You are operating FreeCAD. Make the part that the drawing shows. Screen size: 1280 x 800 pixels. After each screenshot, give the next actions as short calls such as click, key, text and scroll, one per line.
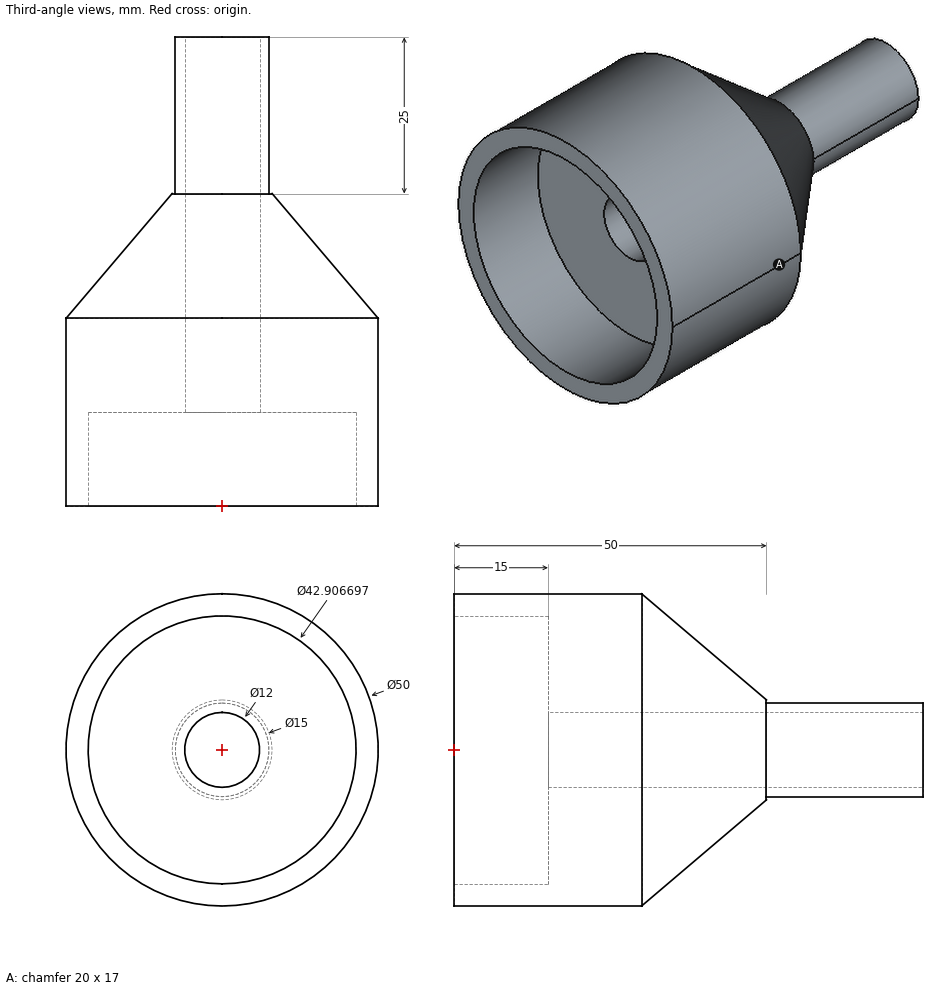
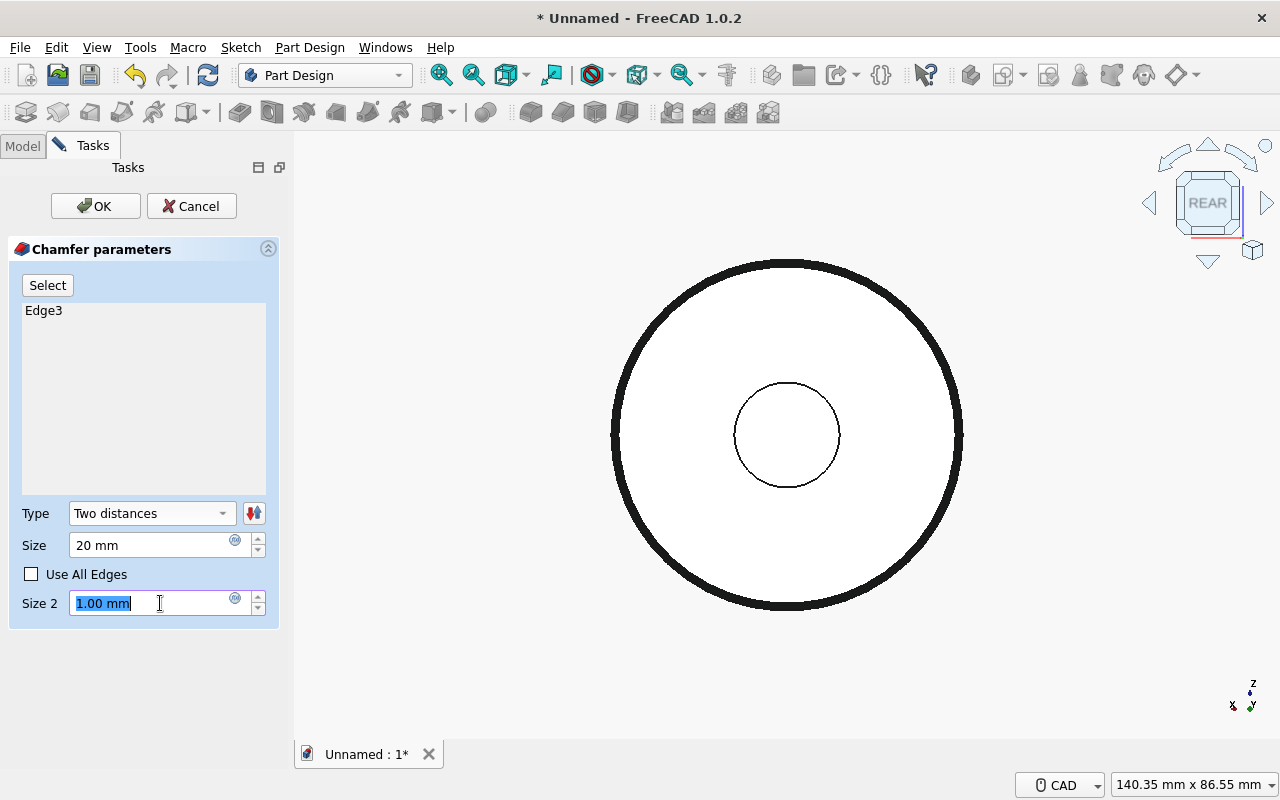
text(17)
key(Tab)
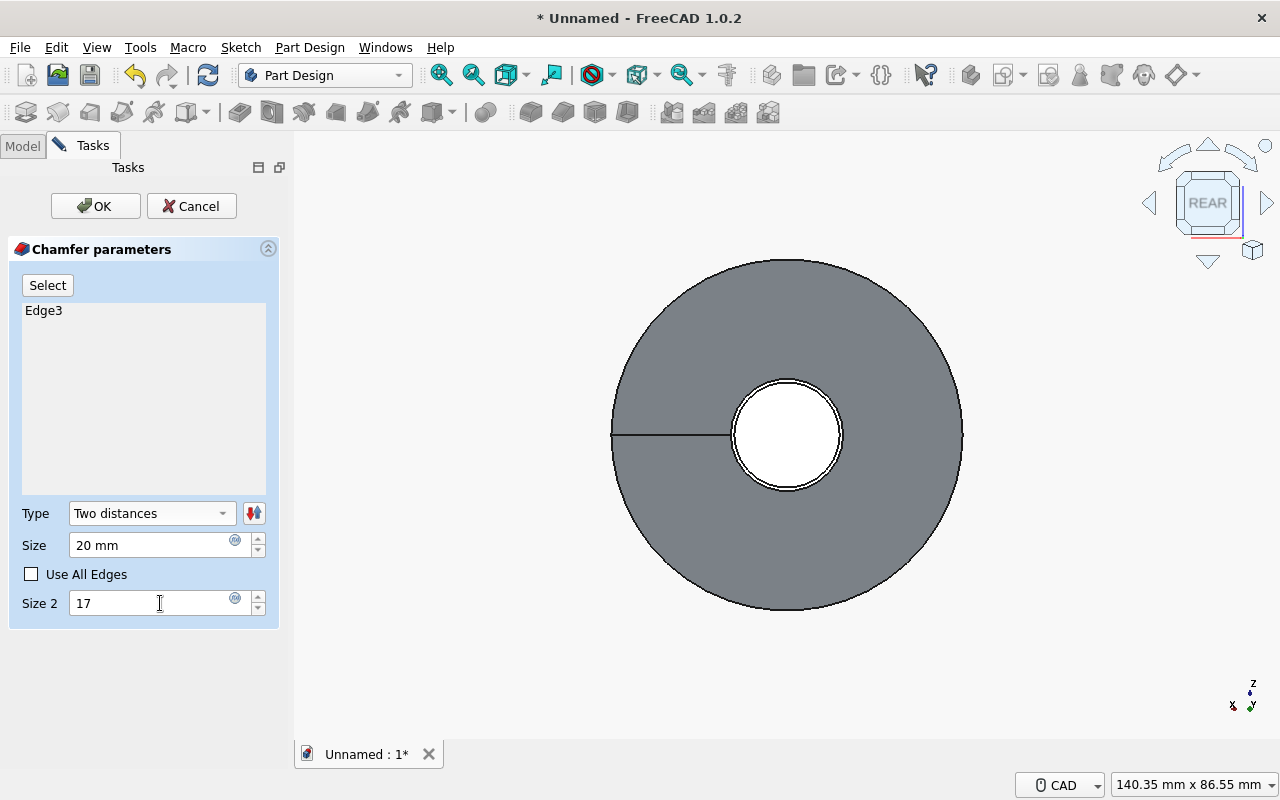
click(96, 206)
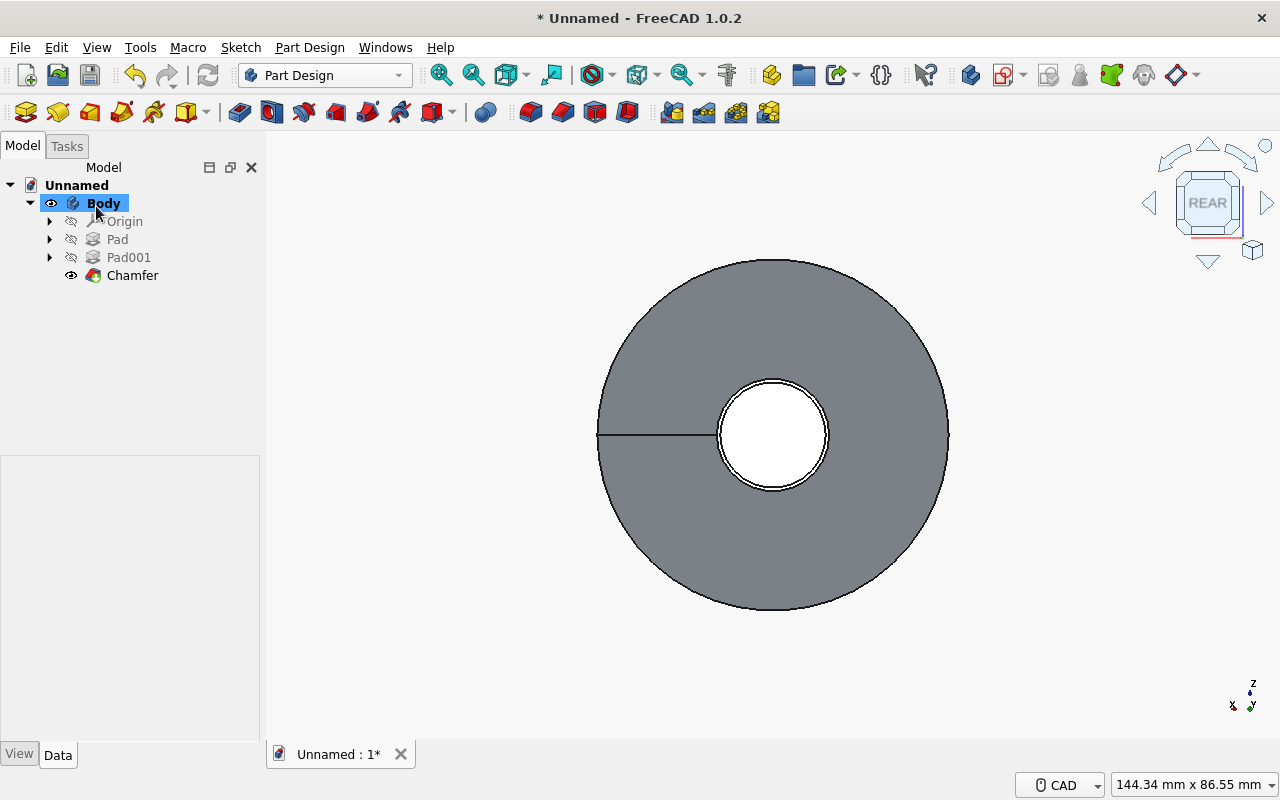
click(773, 434)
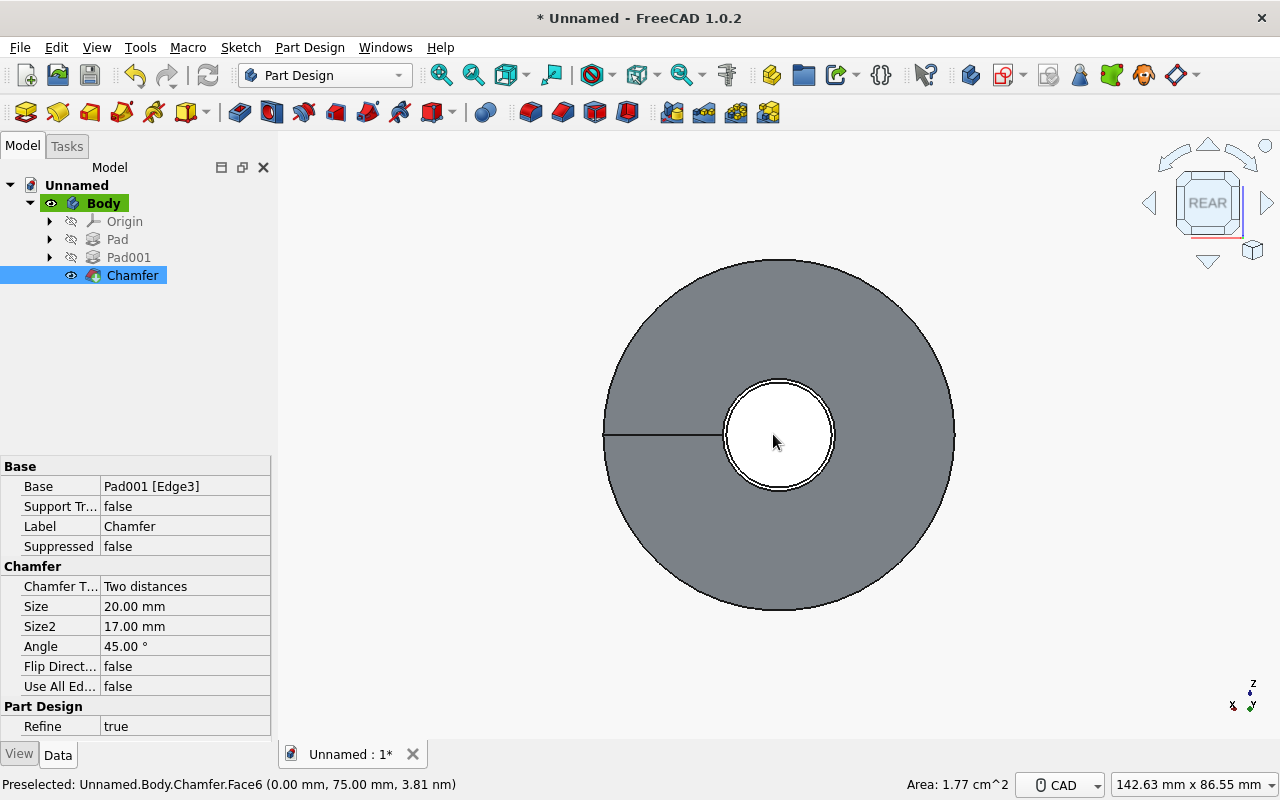
click(1004, 76)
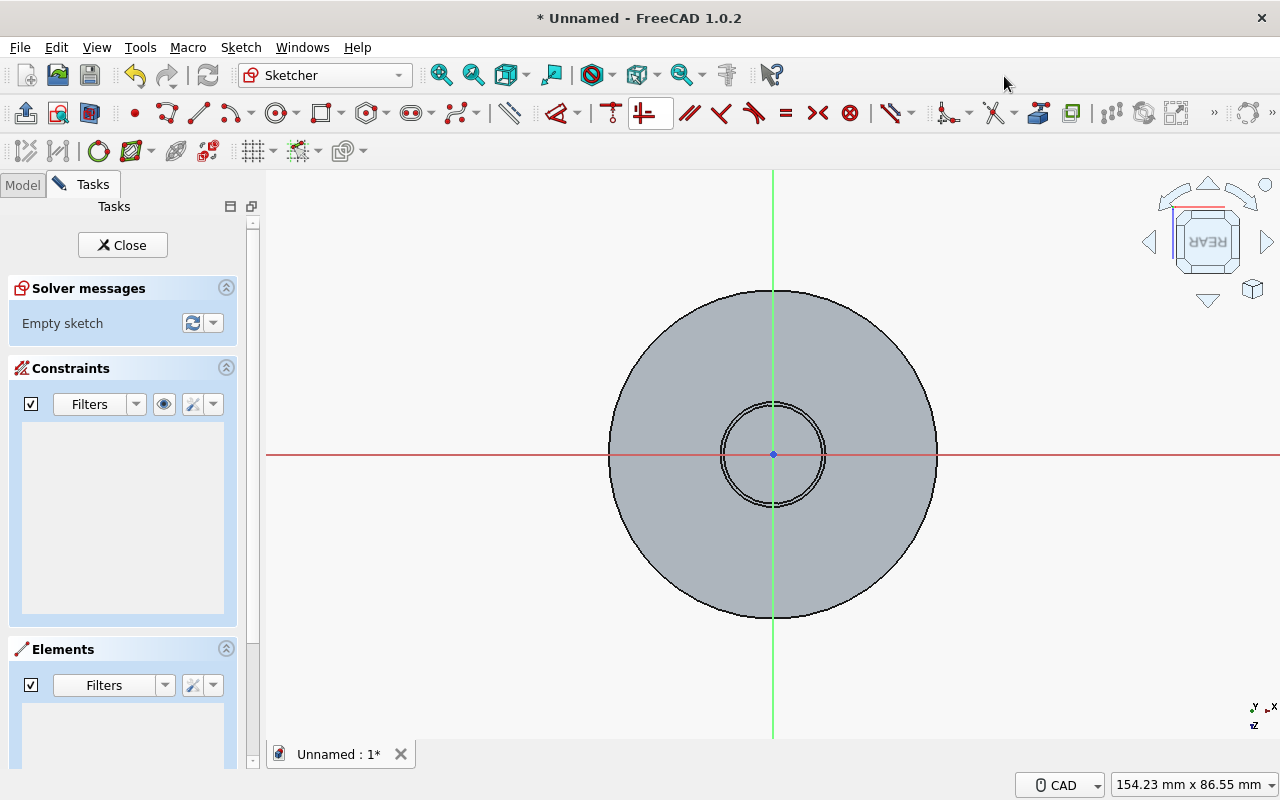
scroll(790, 454, up, 8)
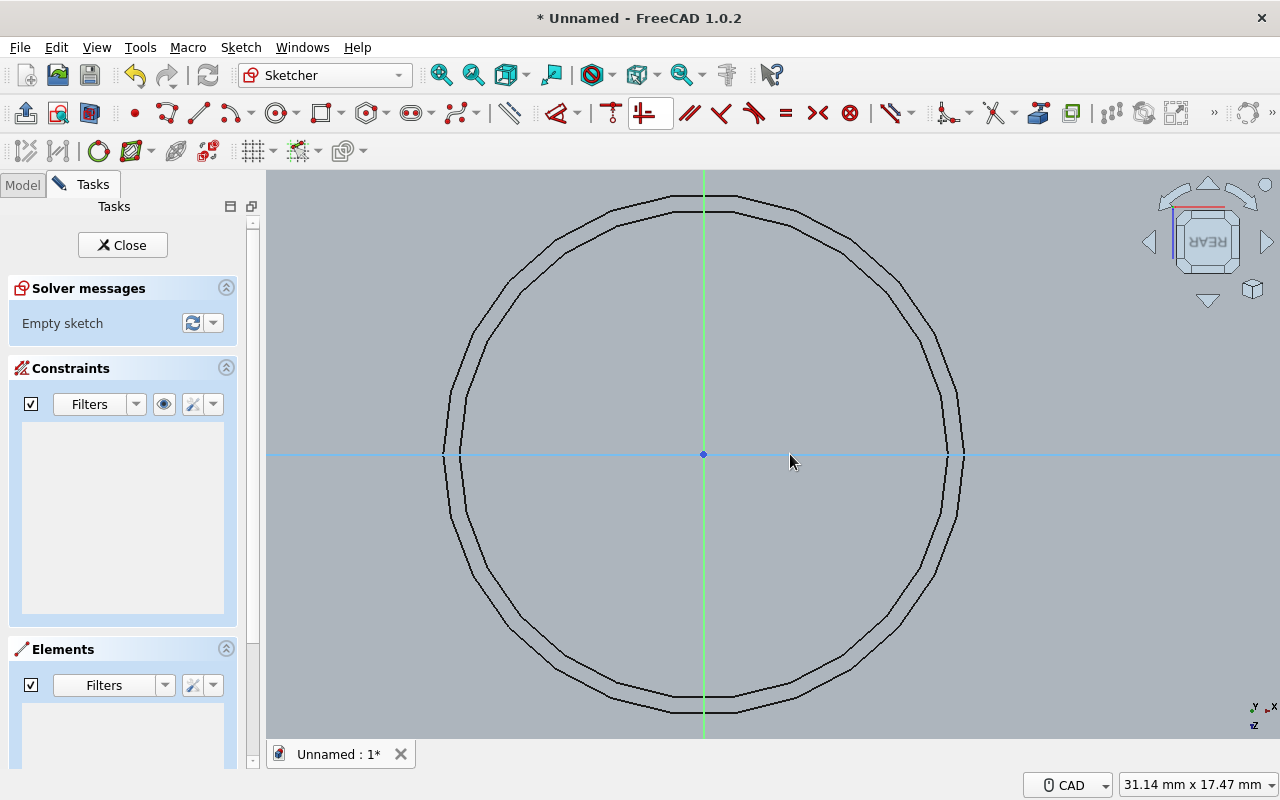
key(g)
key(c)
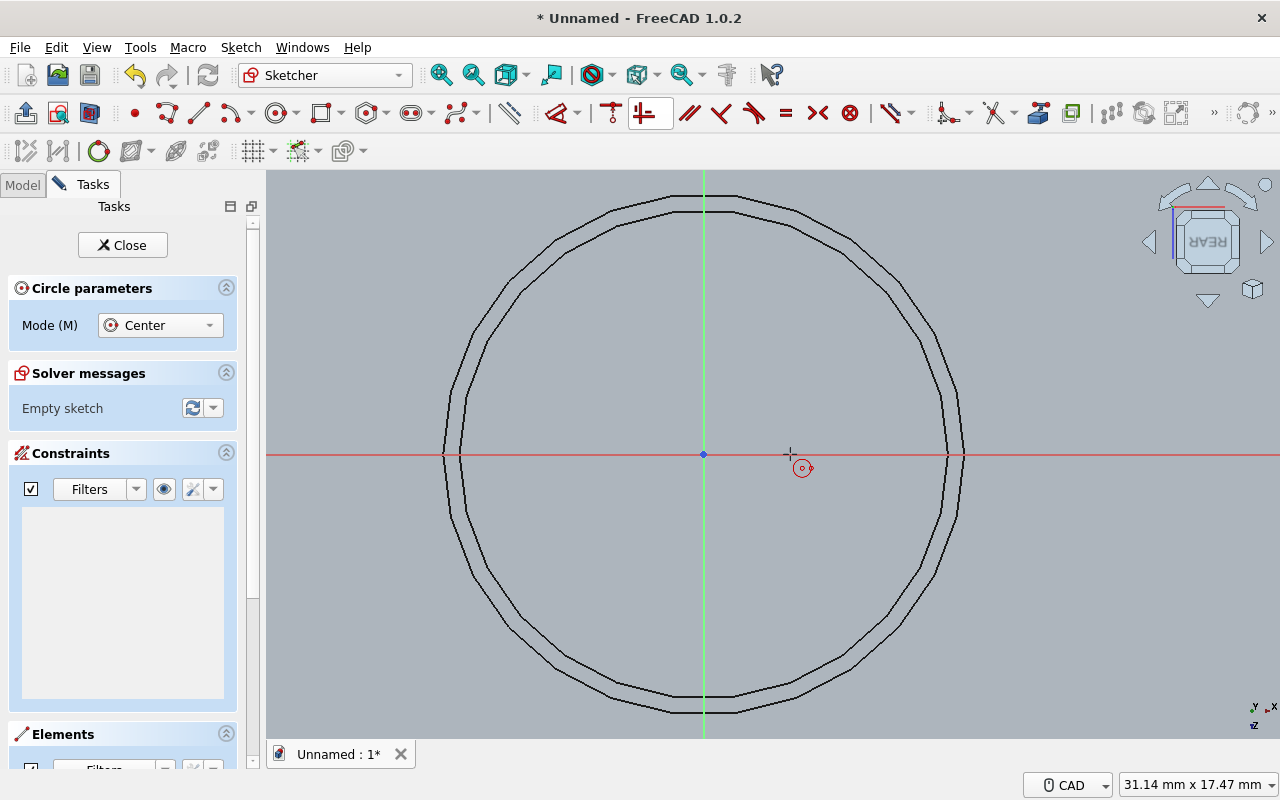
click(704, 454)
move(842, 316)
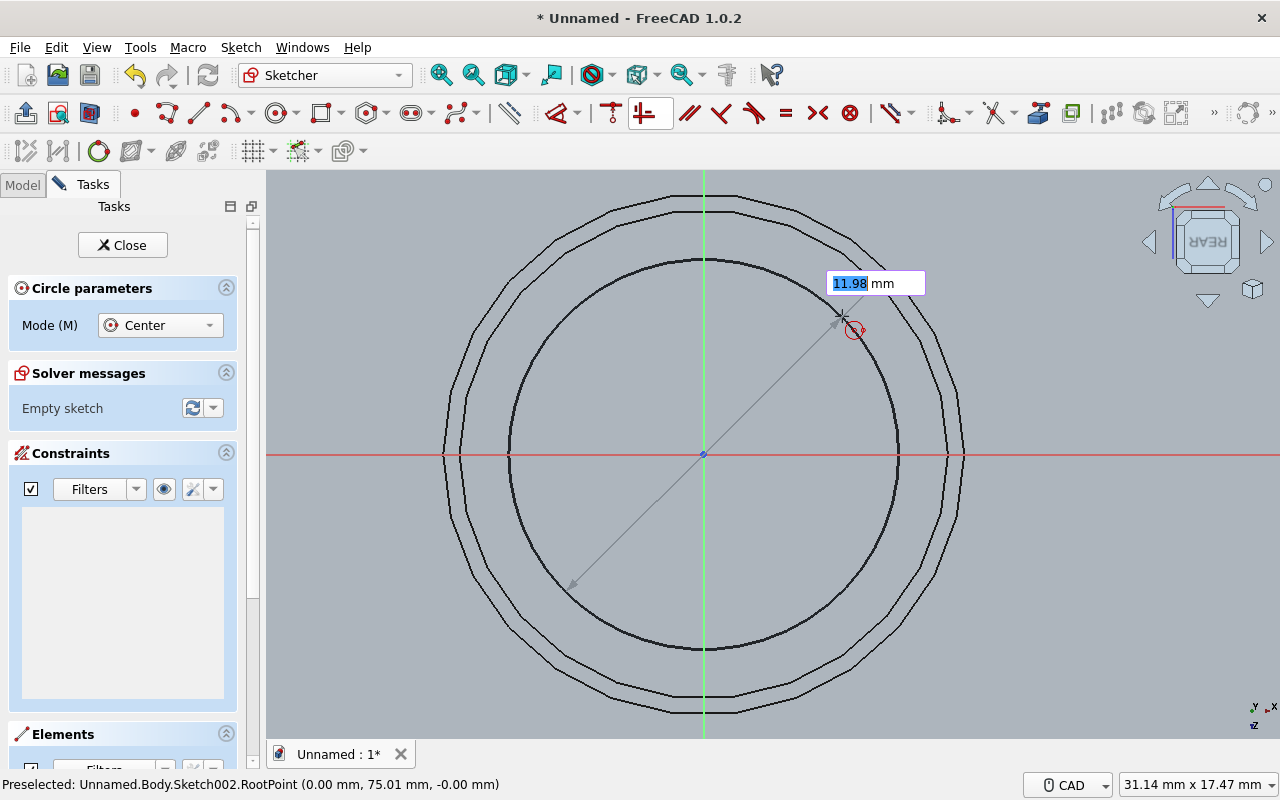
text(12)
key(Return)
key(Escape)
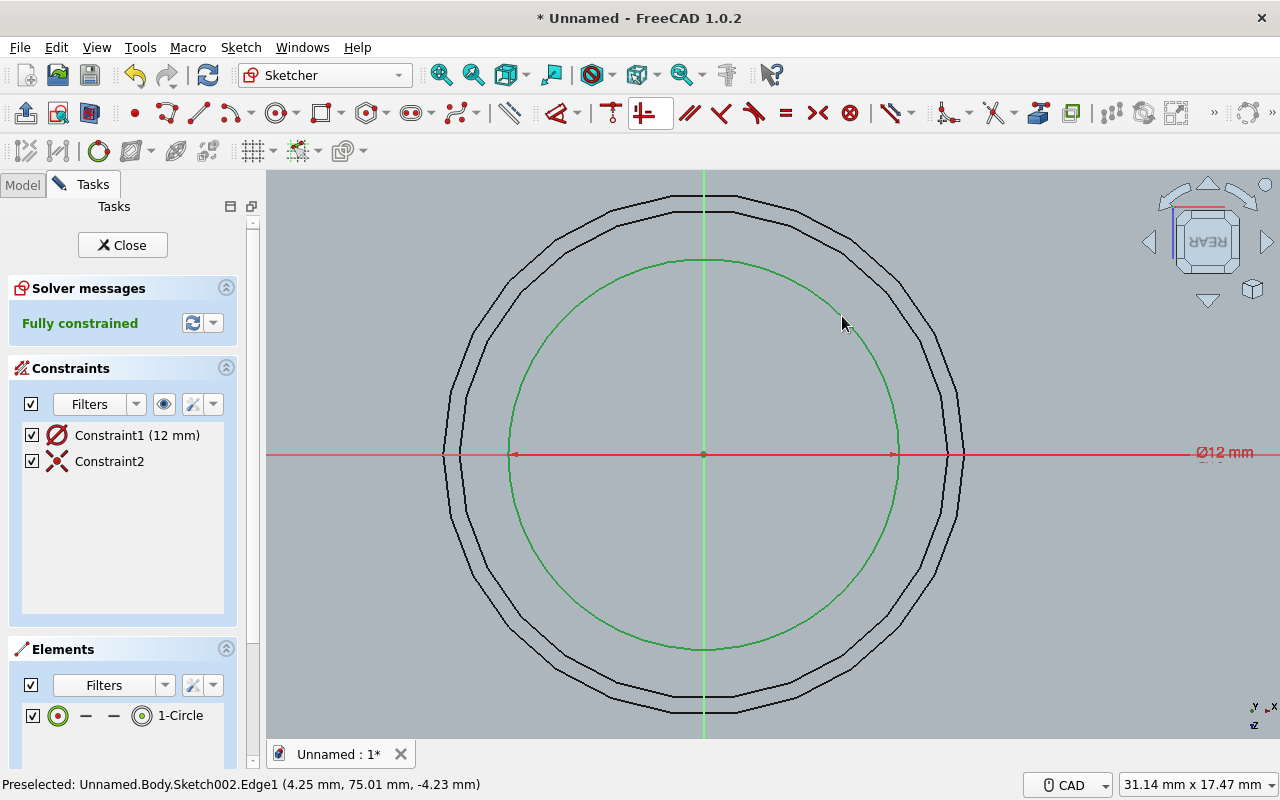
click(123, 245)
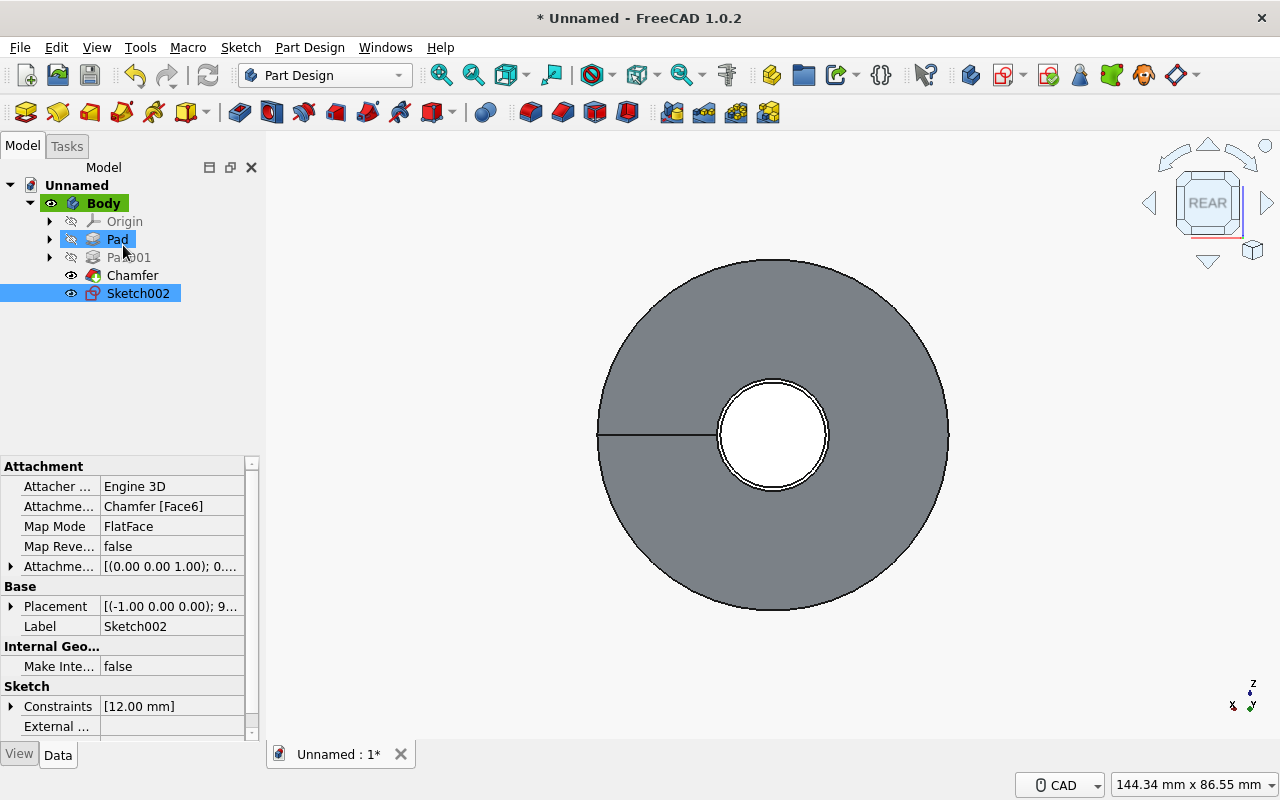
click(240, 112)